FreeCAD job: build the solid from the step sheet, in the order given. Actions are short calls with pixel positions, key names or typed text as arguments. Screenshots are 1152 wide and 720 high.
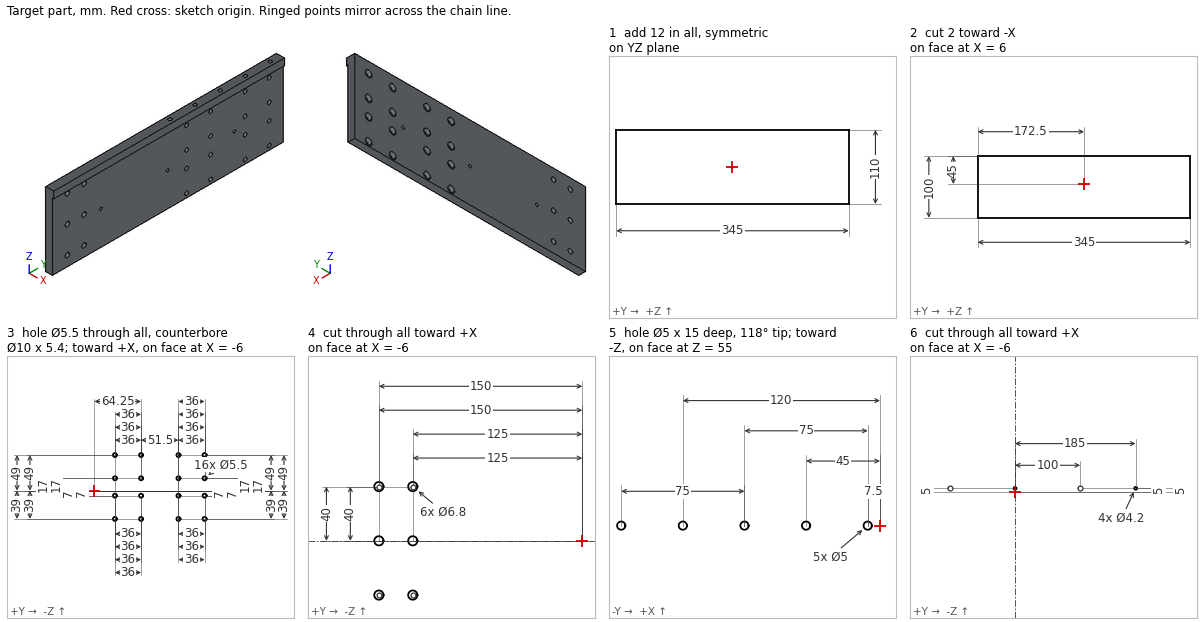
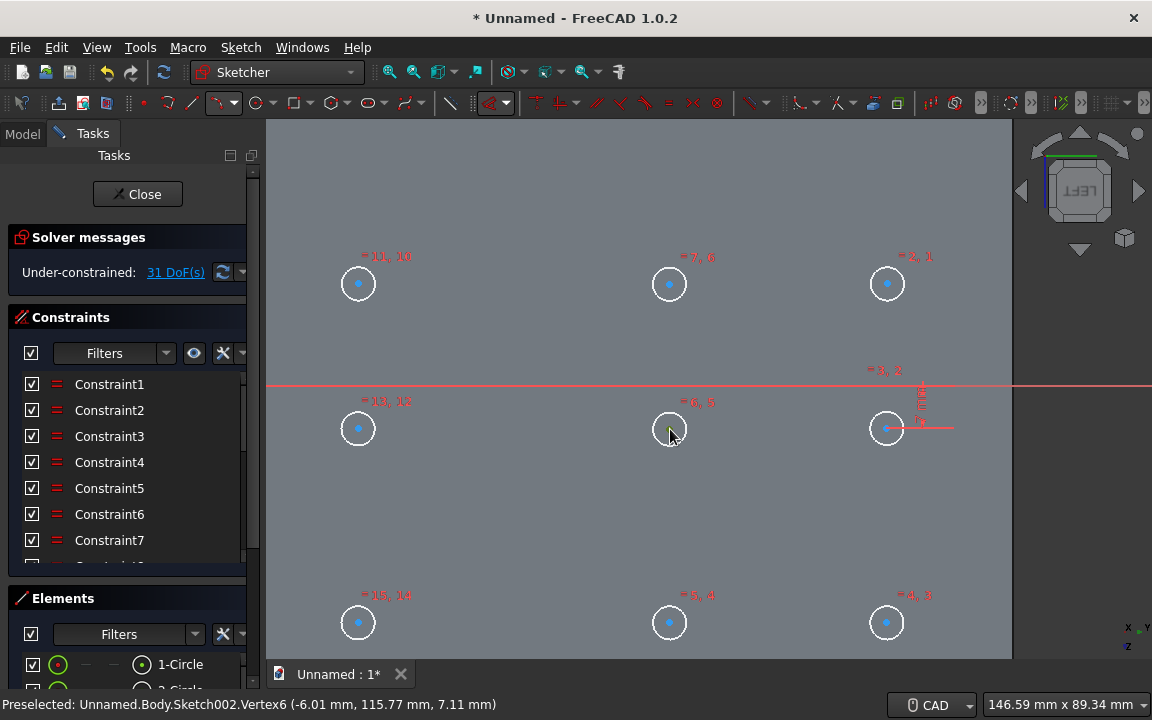
click(508, 104)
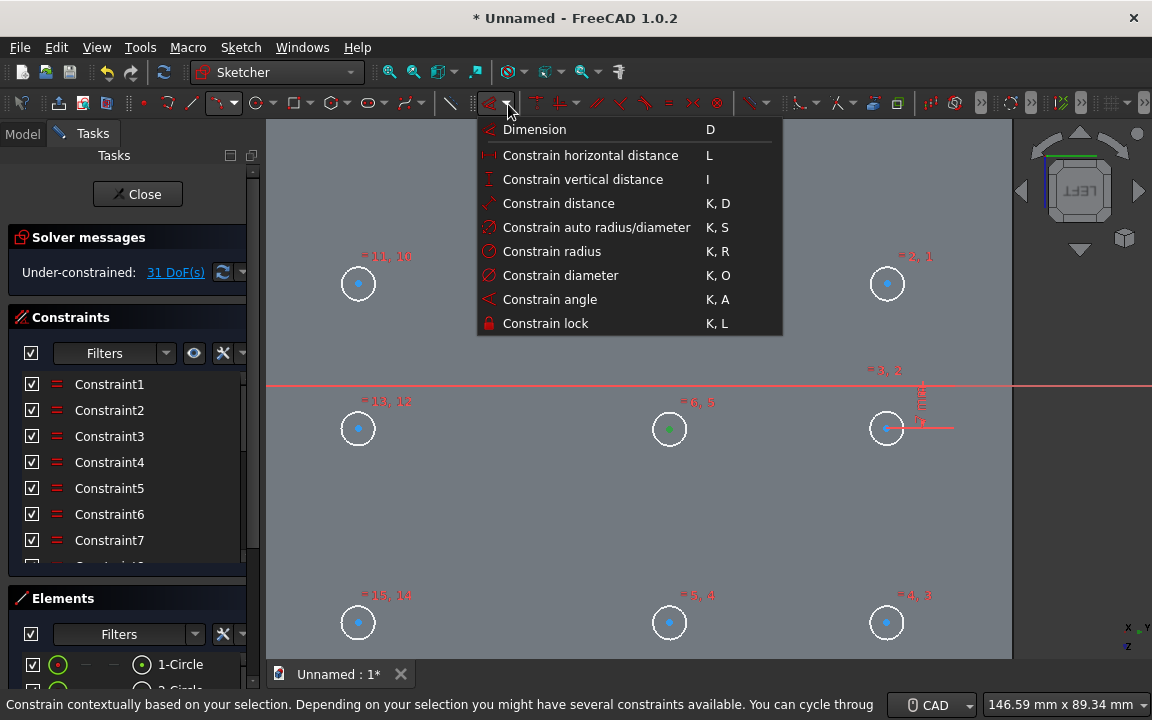
click(630, 179)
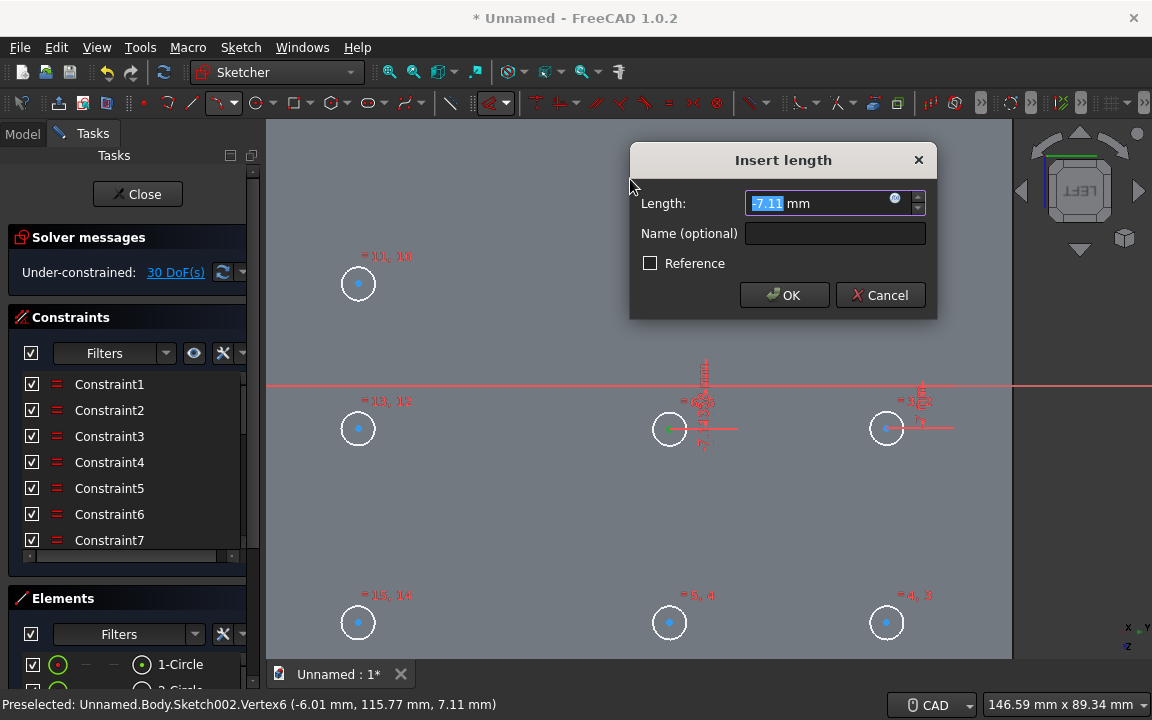
text(-7)
key(Return)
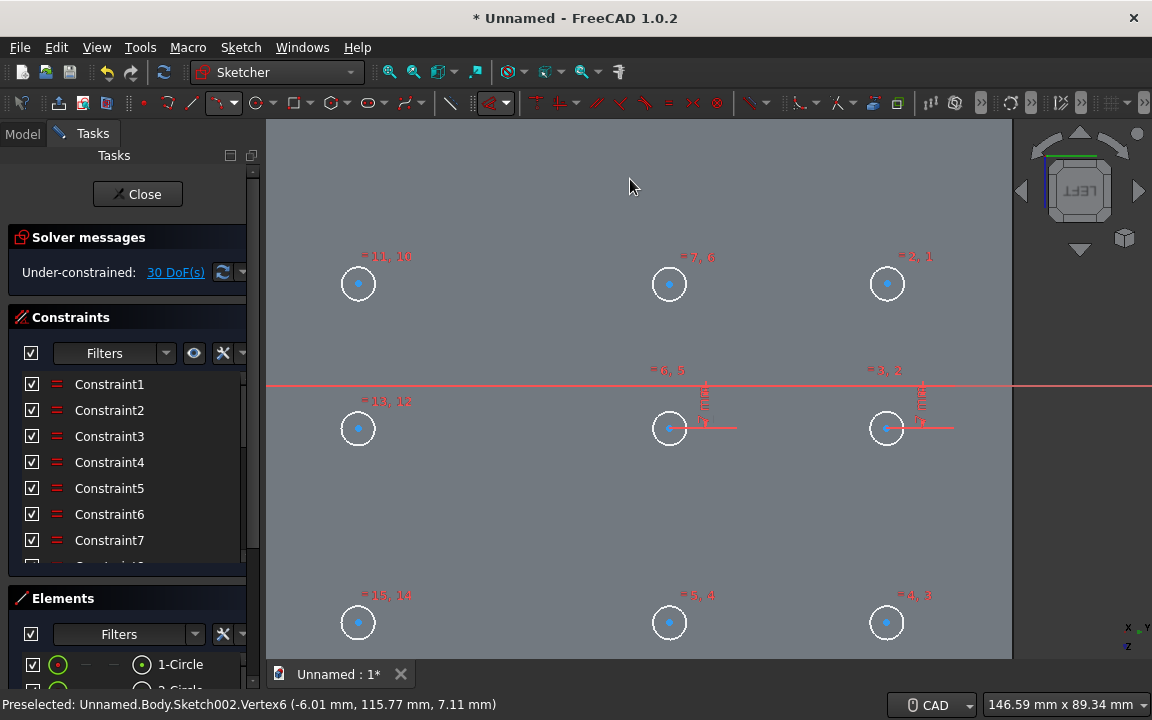
click(358, 429)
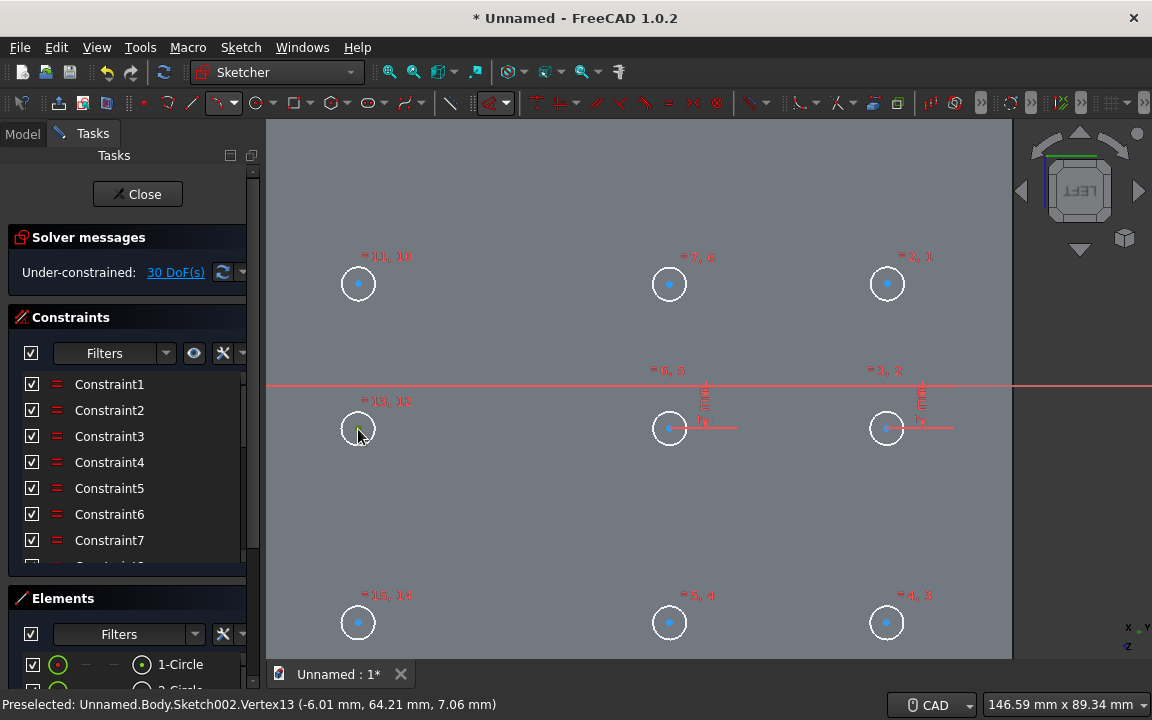
key(i)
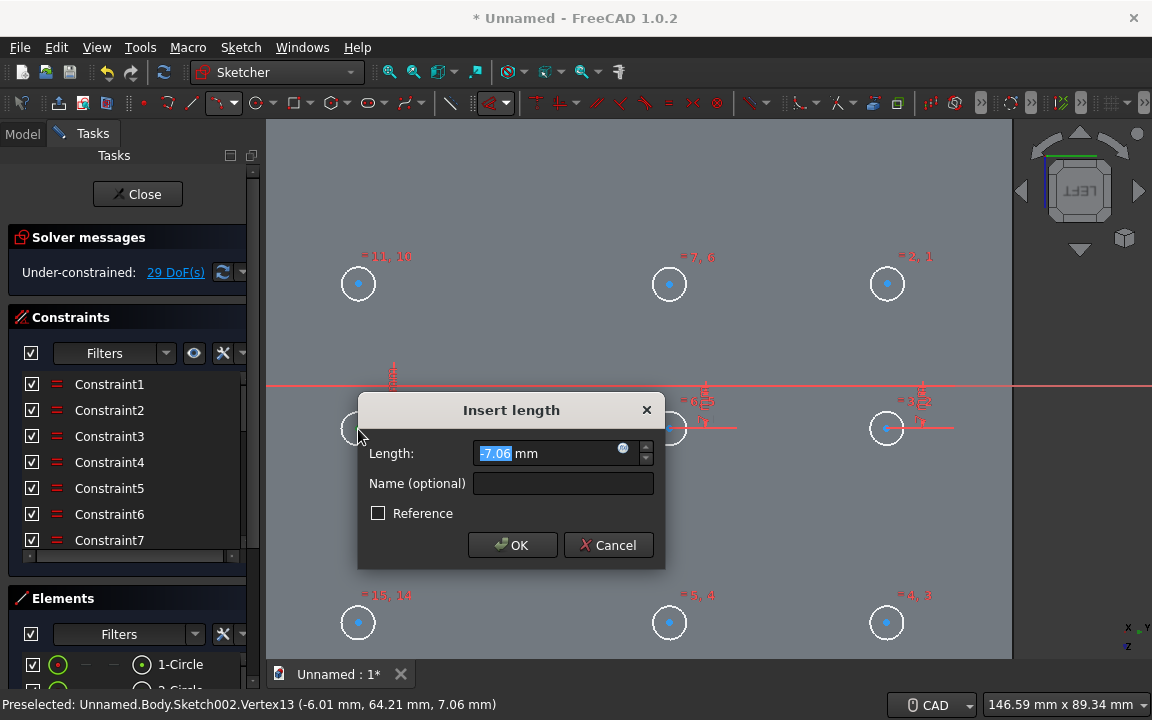
text(-7)
key(Return)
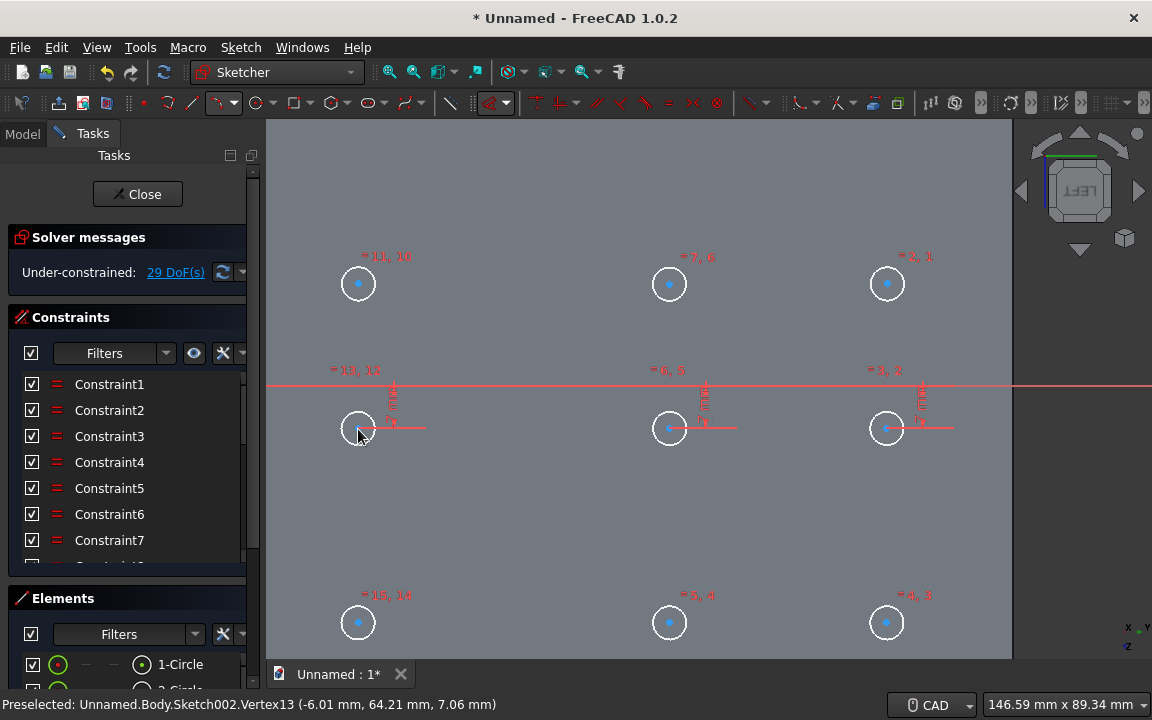
scroll(888, 429, down, 3)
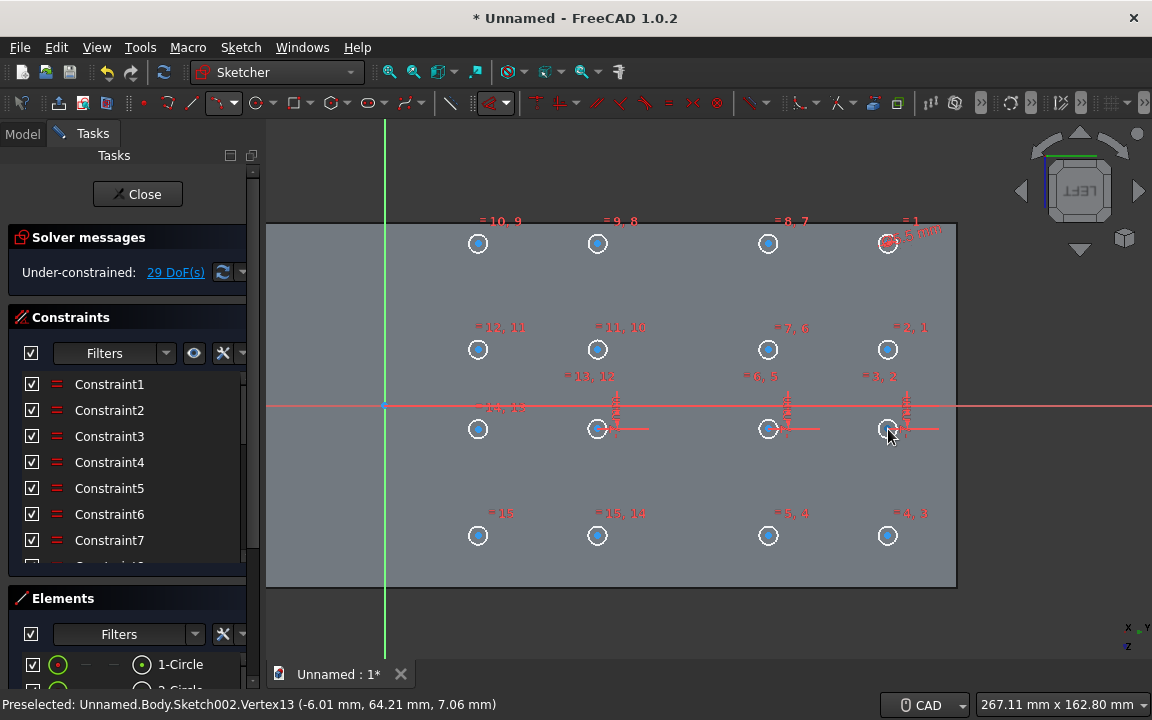
scroll(478, 429, up, 3)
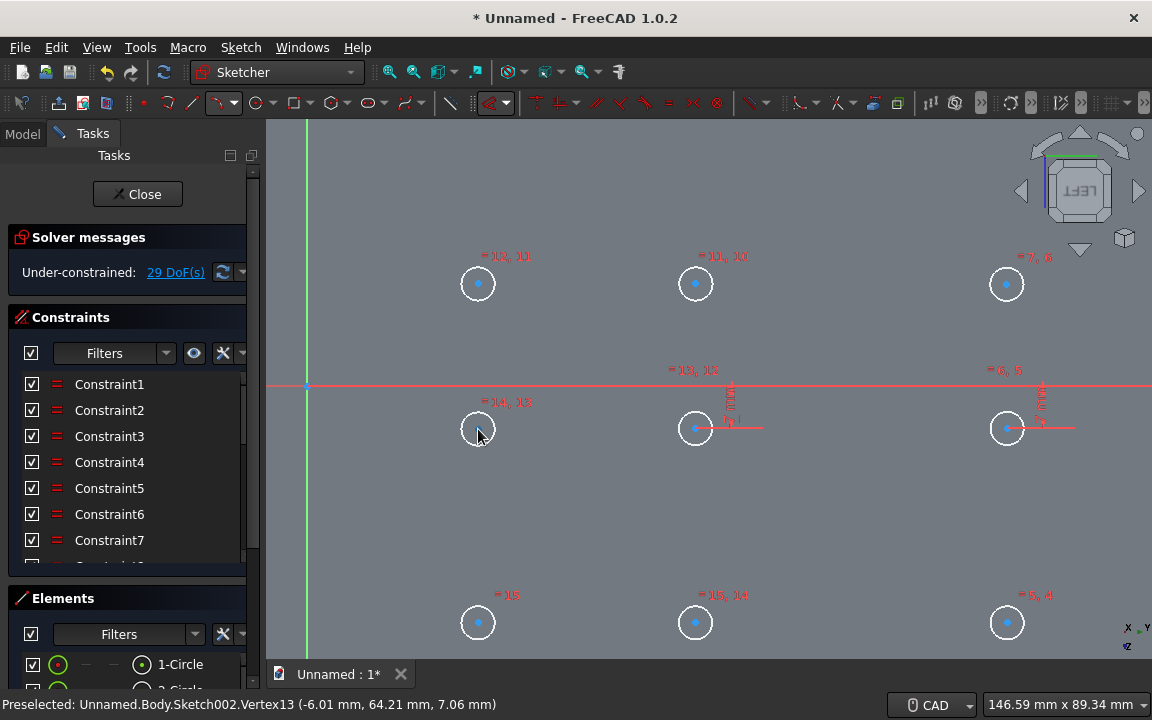
click(478, 429)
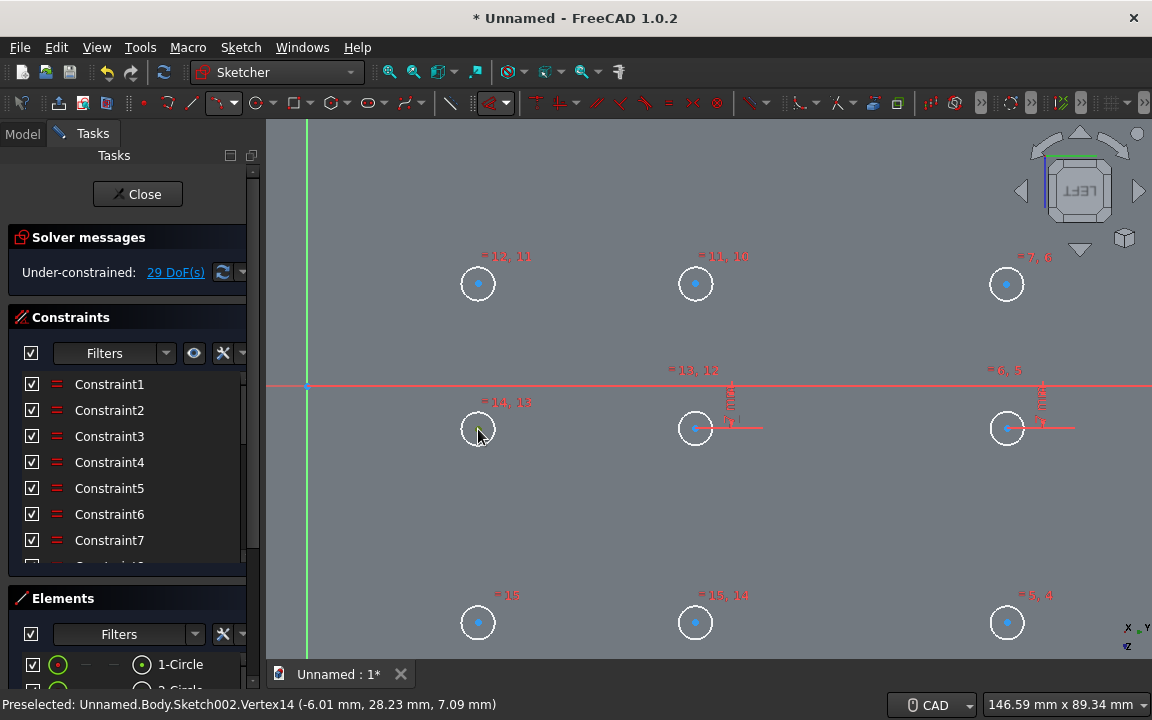
click(508, 104)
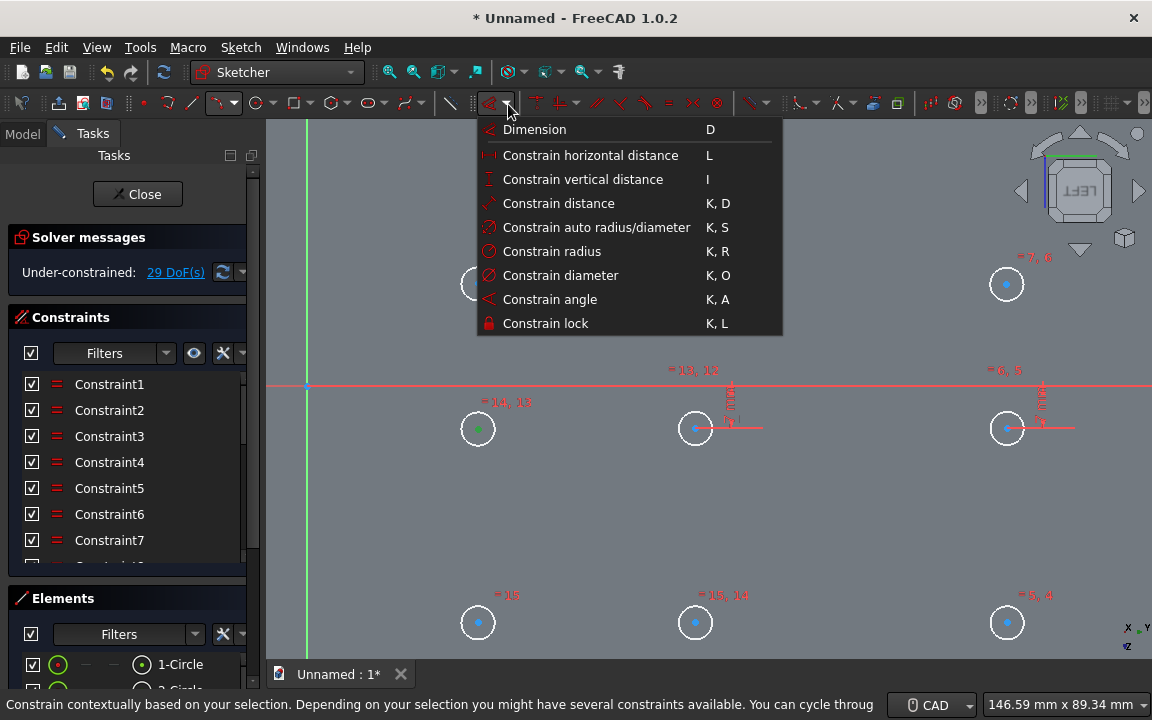
click(630, 179)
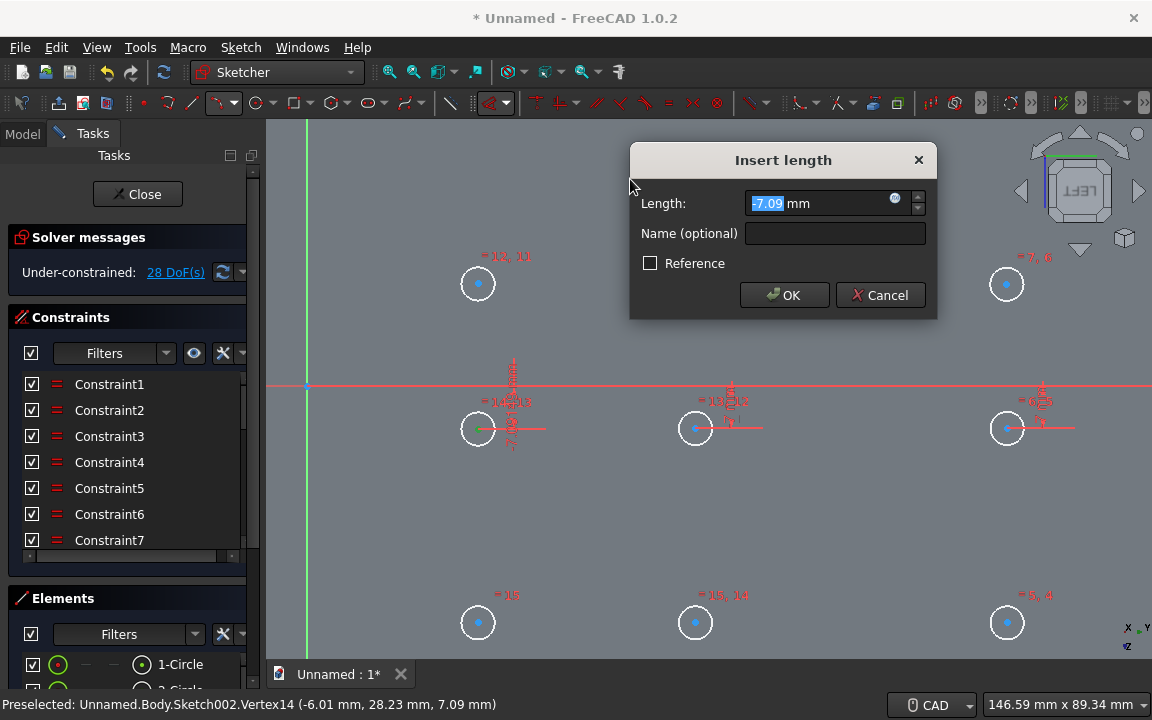
text(-7)
key(Return)